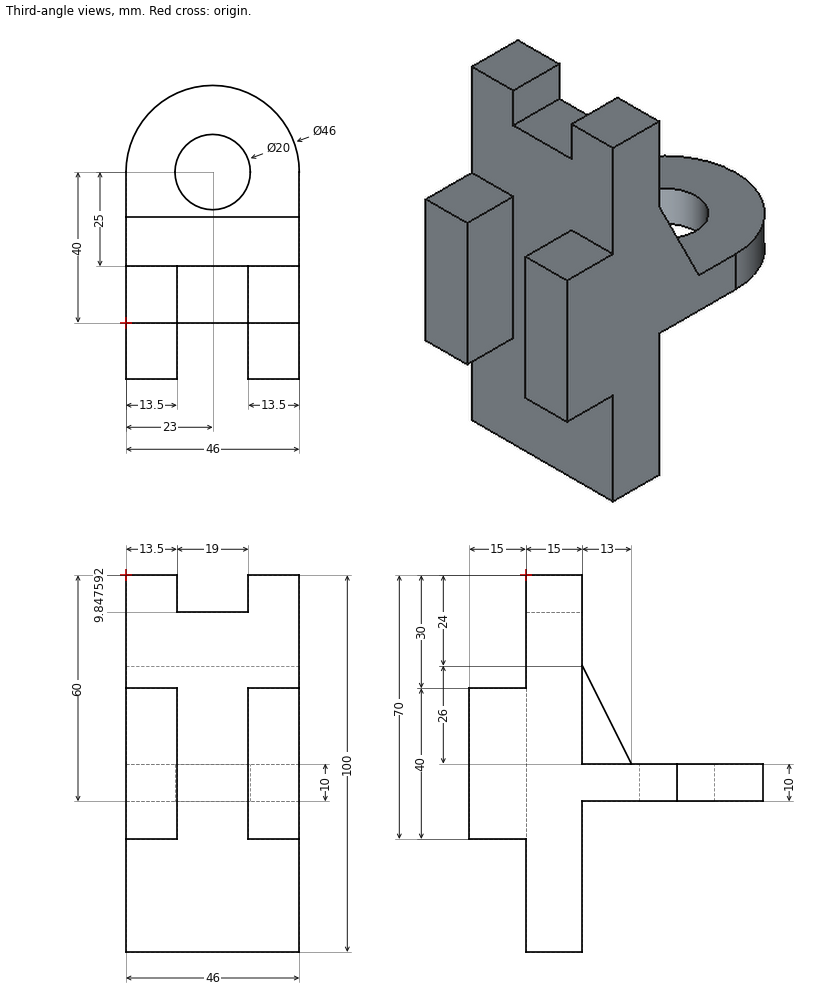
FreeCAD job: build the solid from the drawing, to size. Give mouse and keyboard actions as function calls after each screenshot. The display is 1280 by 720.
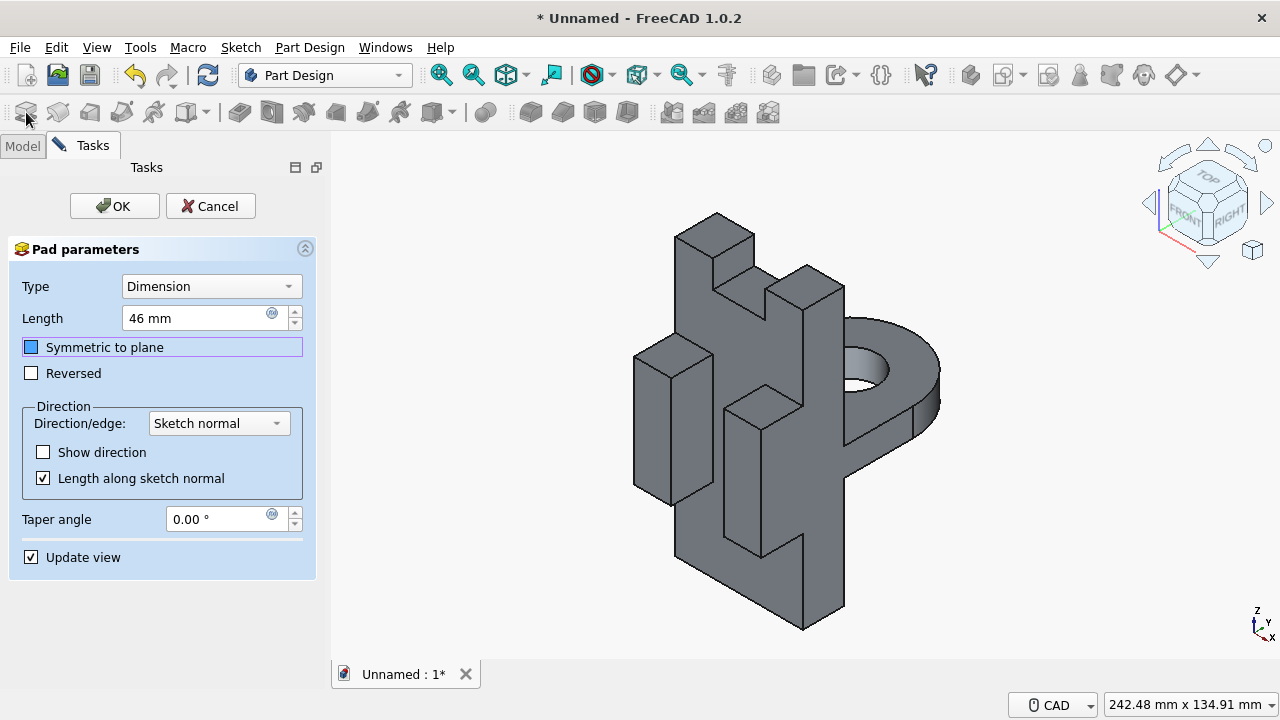
click(30, 373)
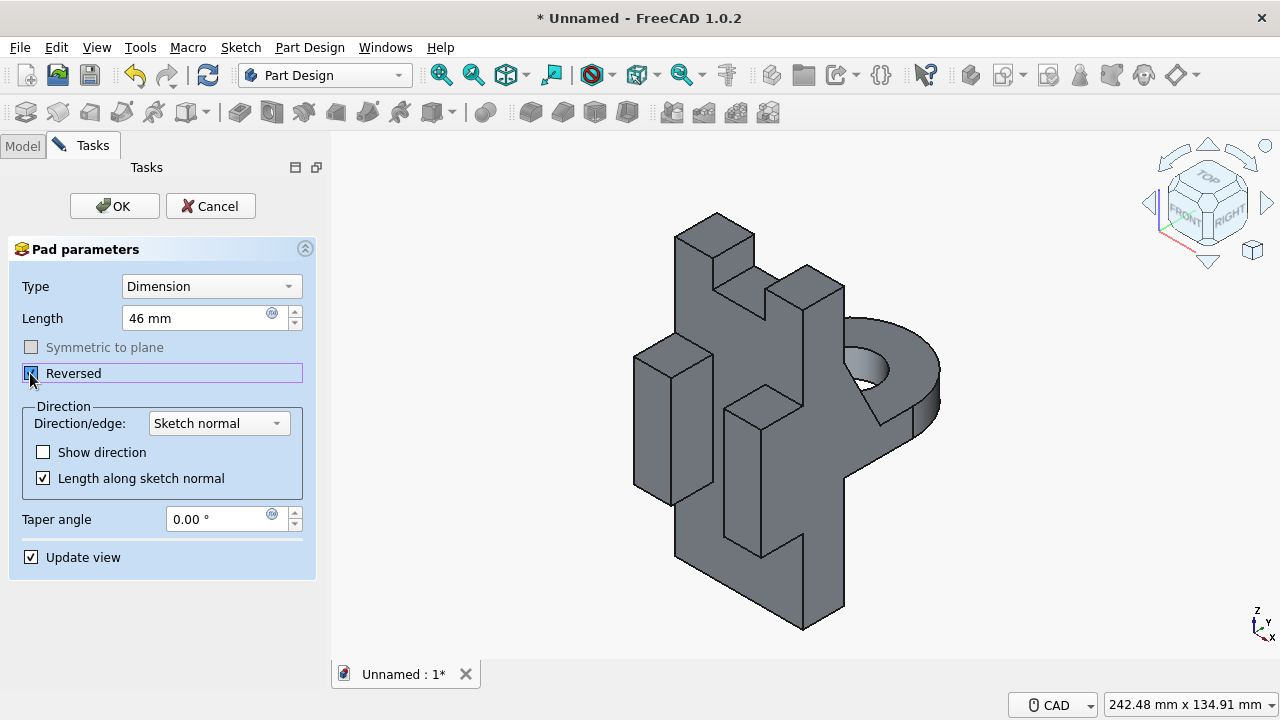
click(115, 206)